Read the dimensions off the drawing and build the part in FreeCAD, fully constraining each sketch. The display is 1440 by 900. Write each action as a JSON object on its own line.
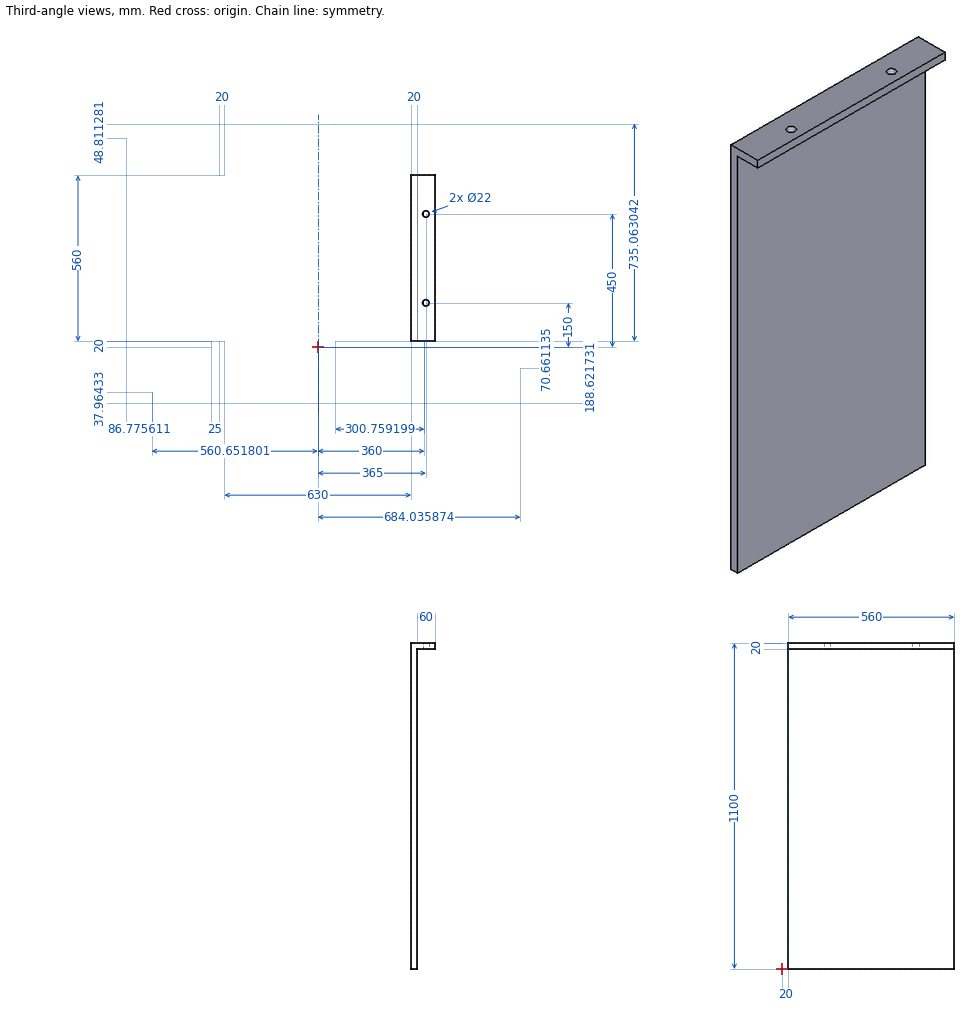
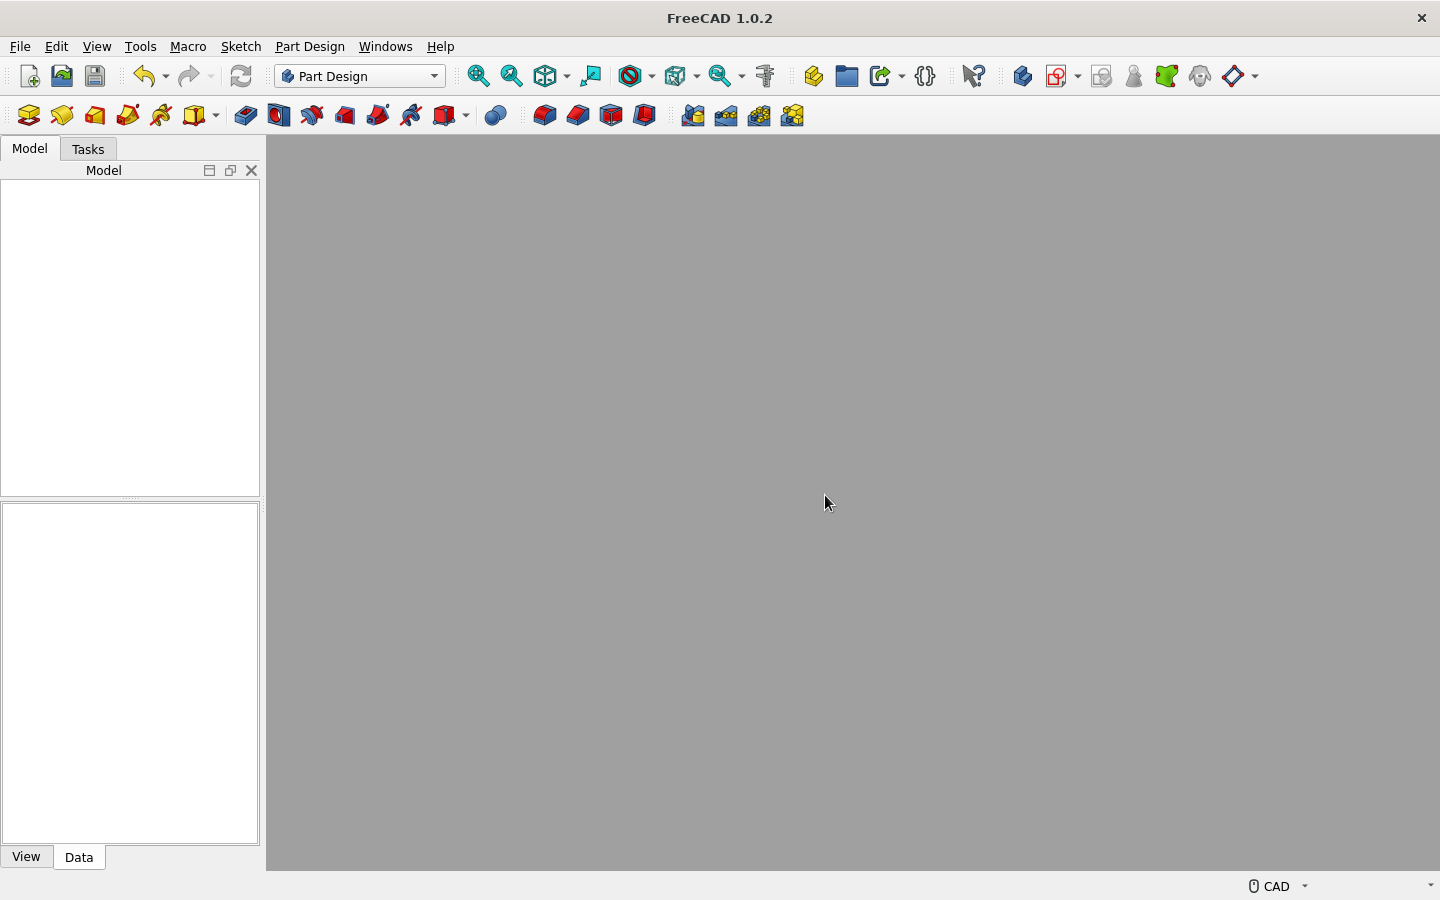
{"action": "left_click", "coordinate": [29, 76]}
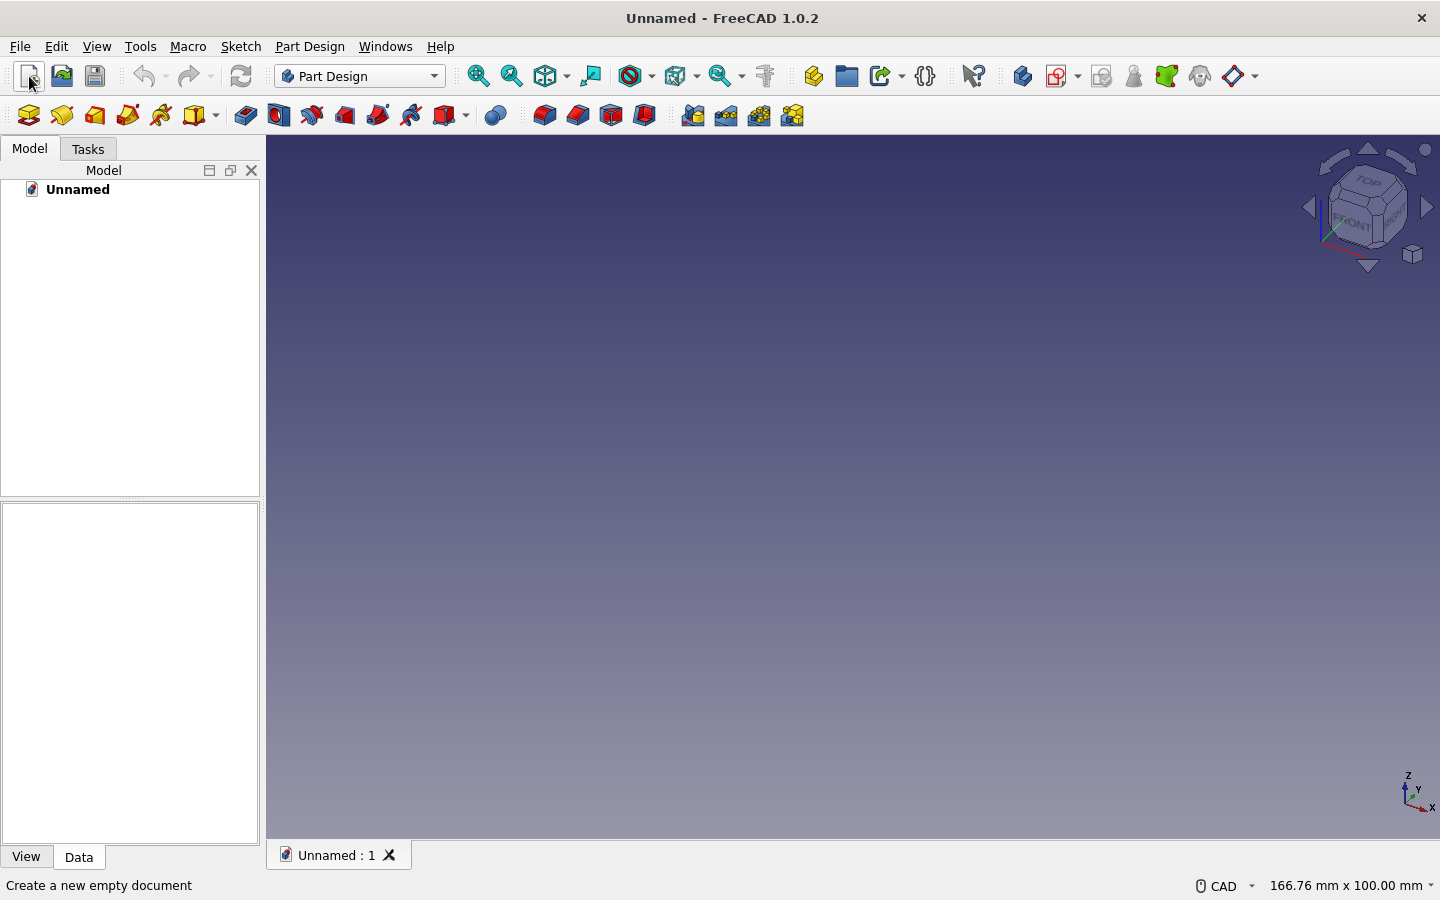
{"action": "left_click", "coordinate": [1056, 76]}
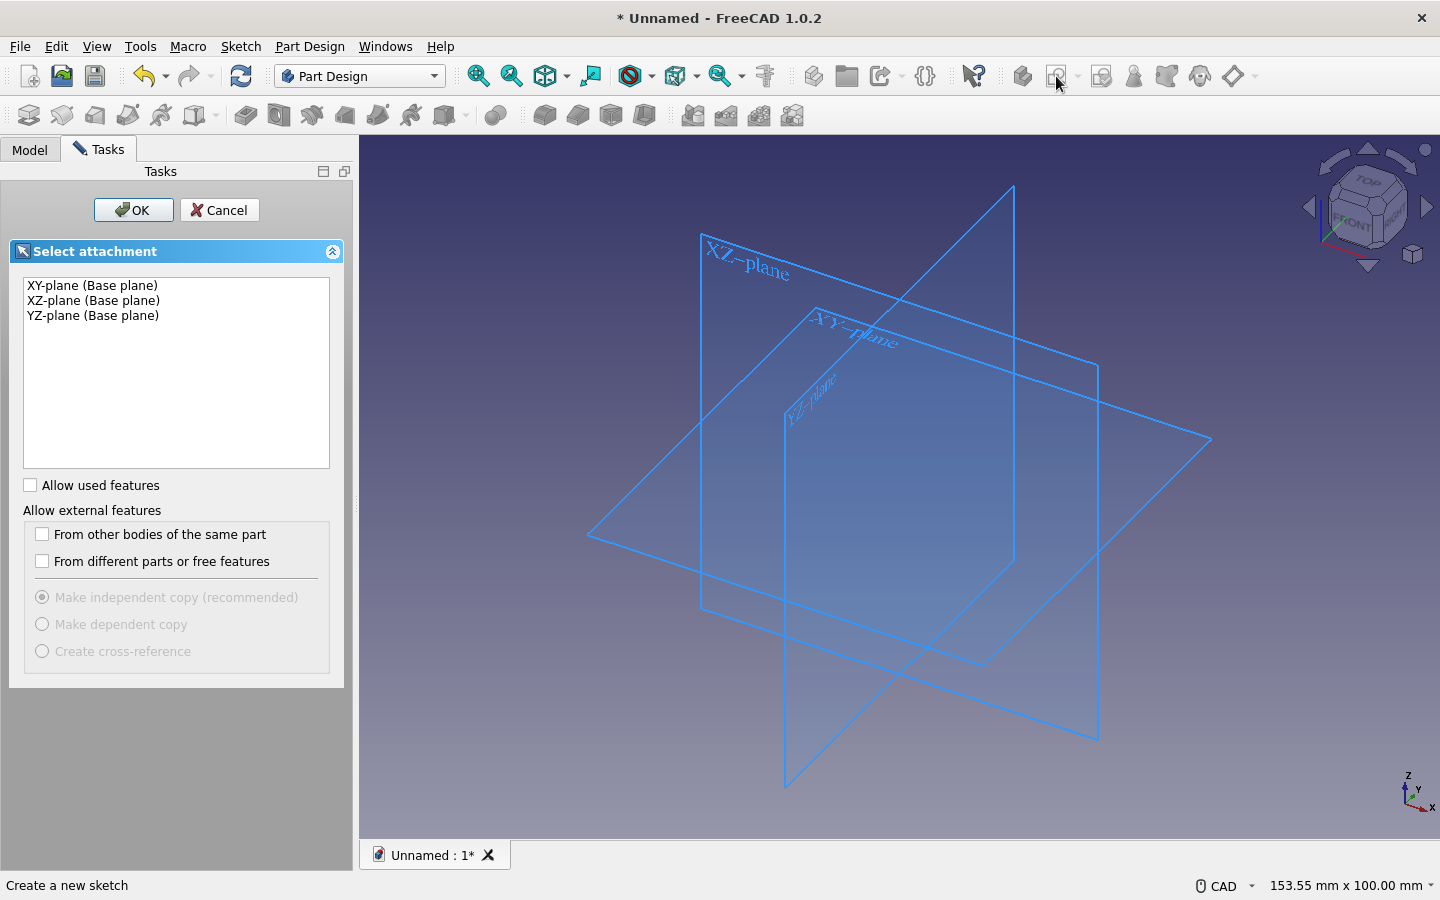
{"action": "left_click", "coordinate": [84, 286]}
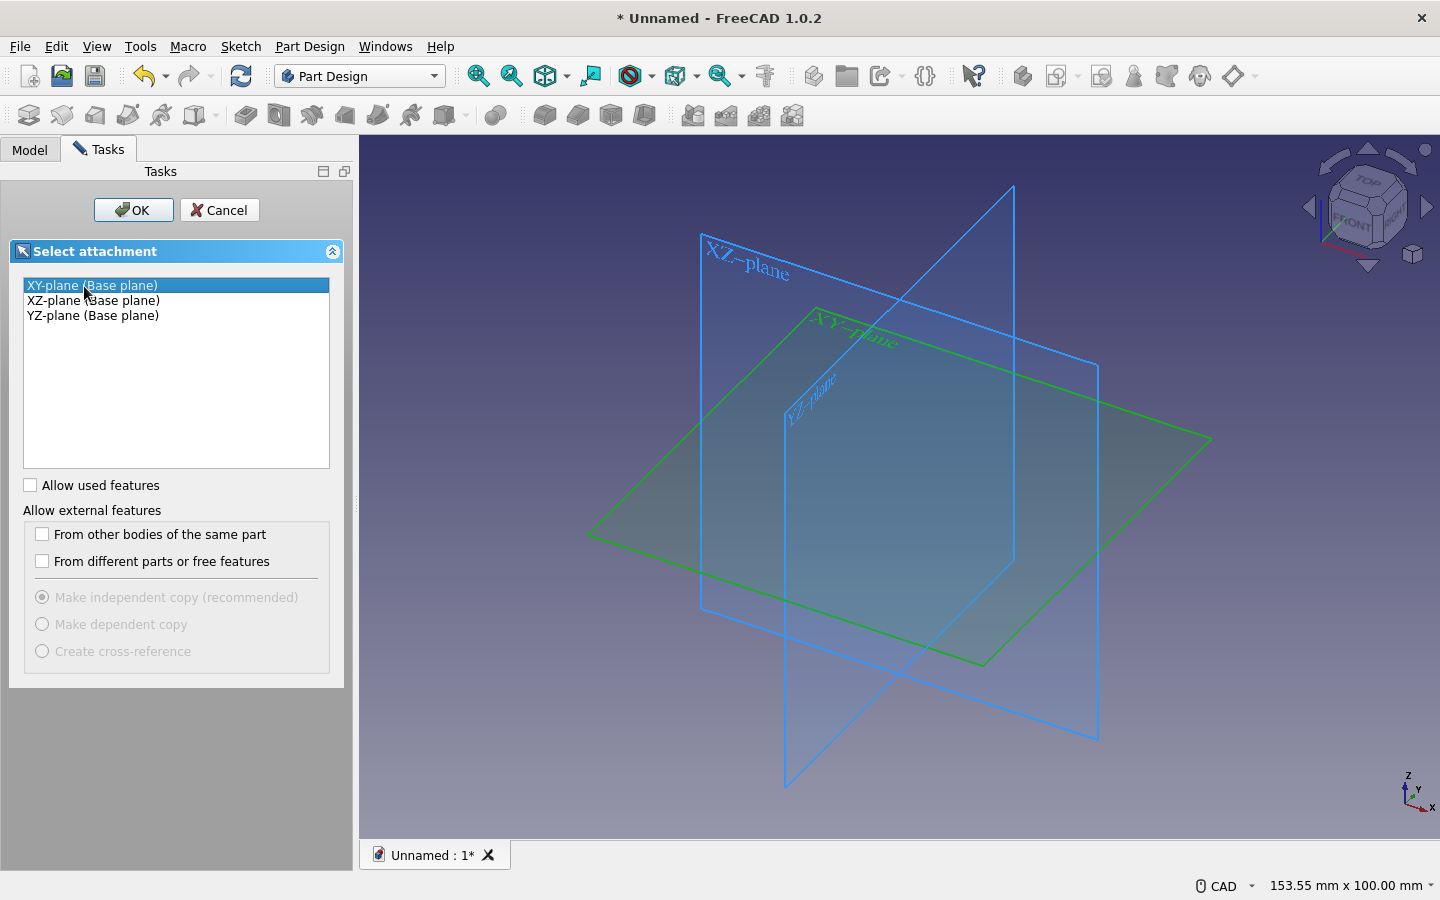
{"action": "left_click", "coordinate": [134, 210]}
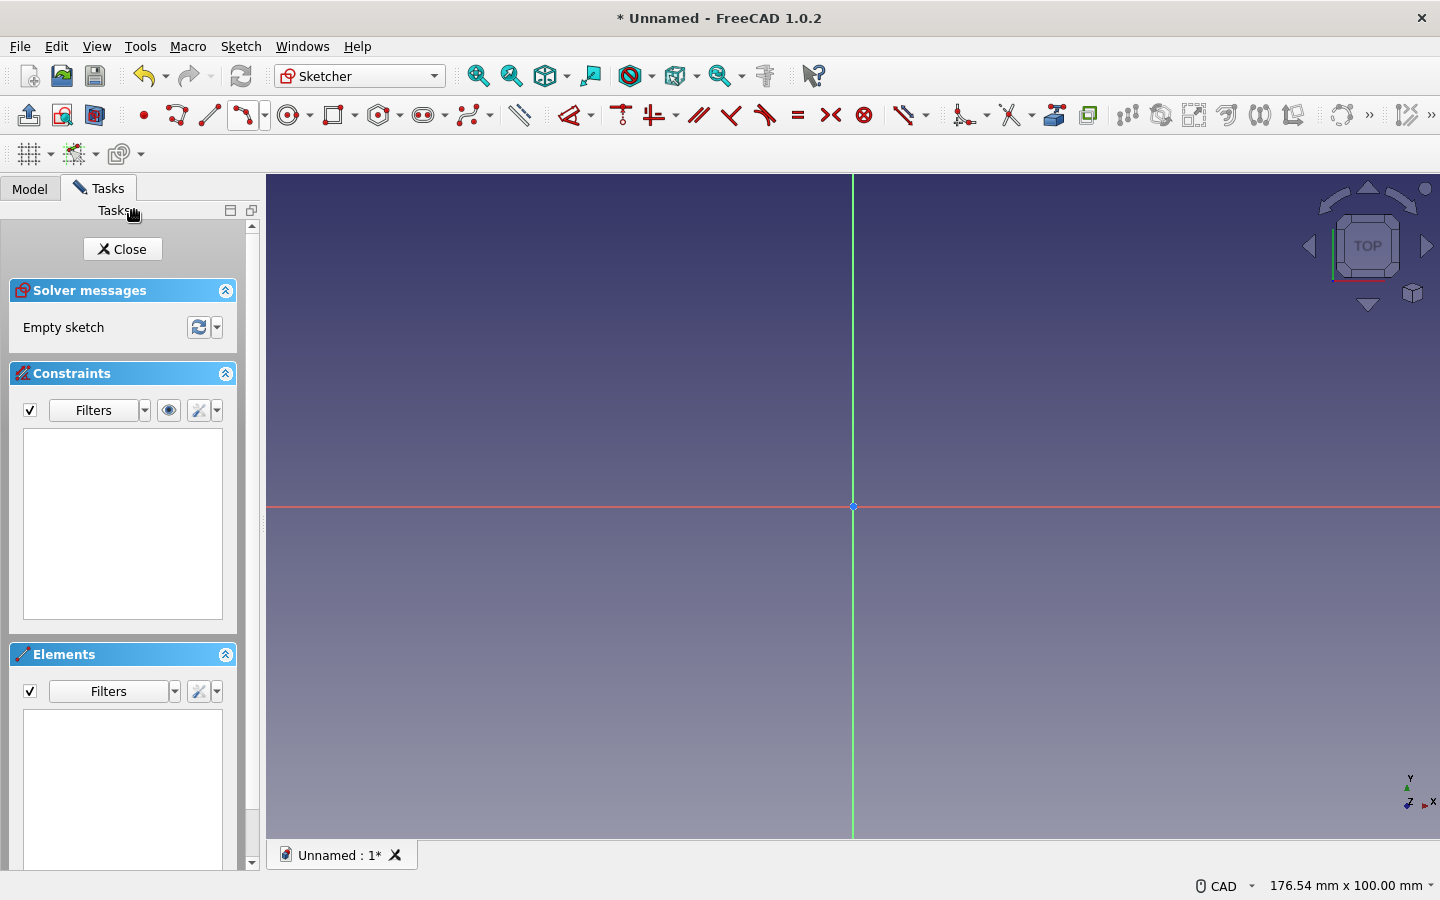
{"action": "scroll", "coordinate": [776, 747], "scroll_direction": "down", "scroll_amount": 11}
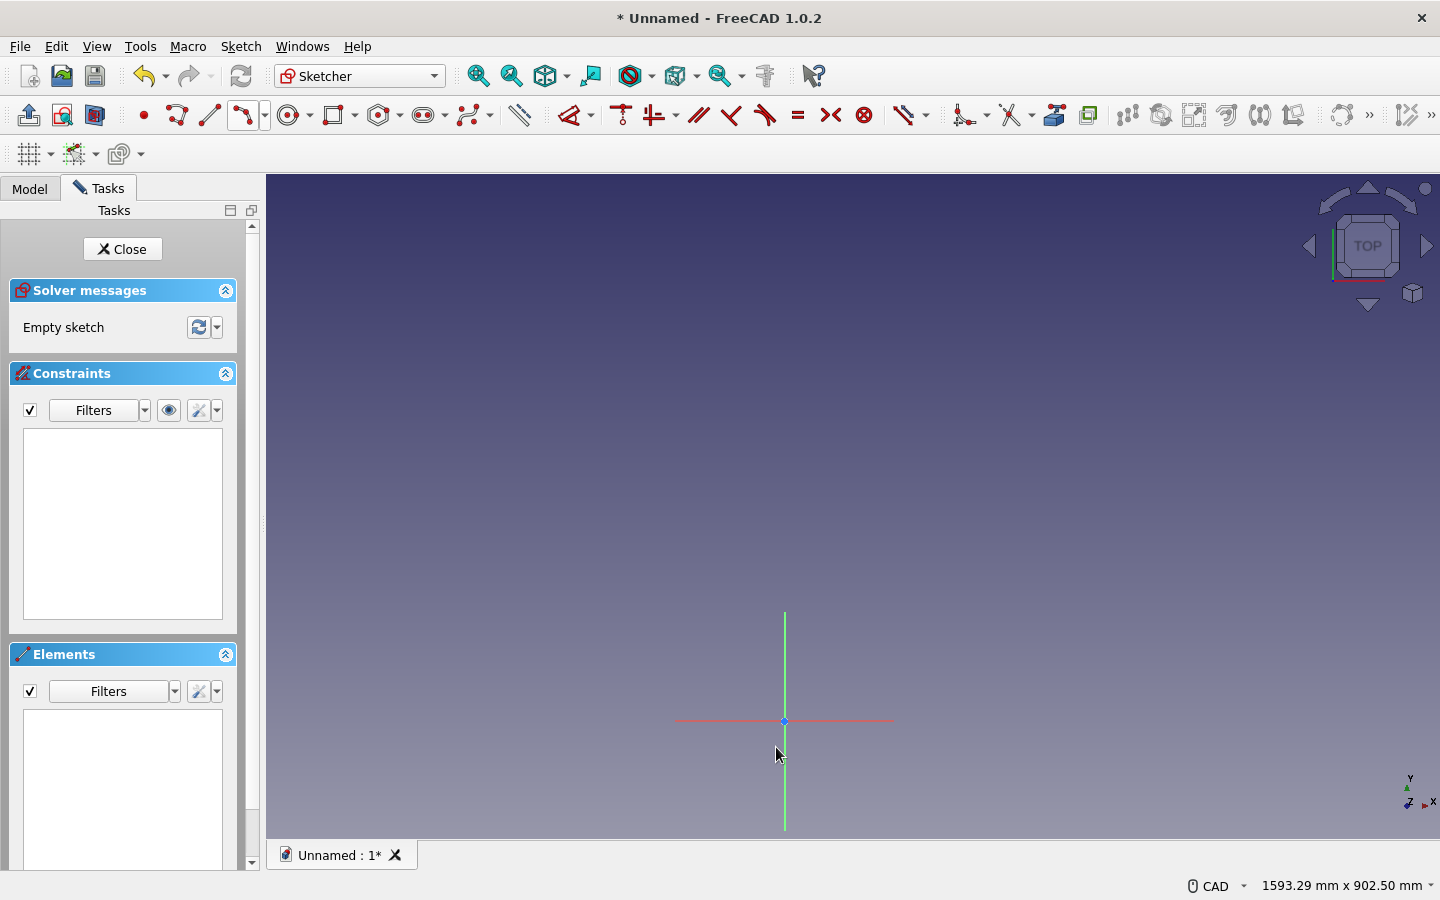
{"action": "left_click", "coordinate": [177, 116]}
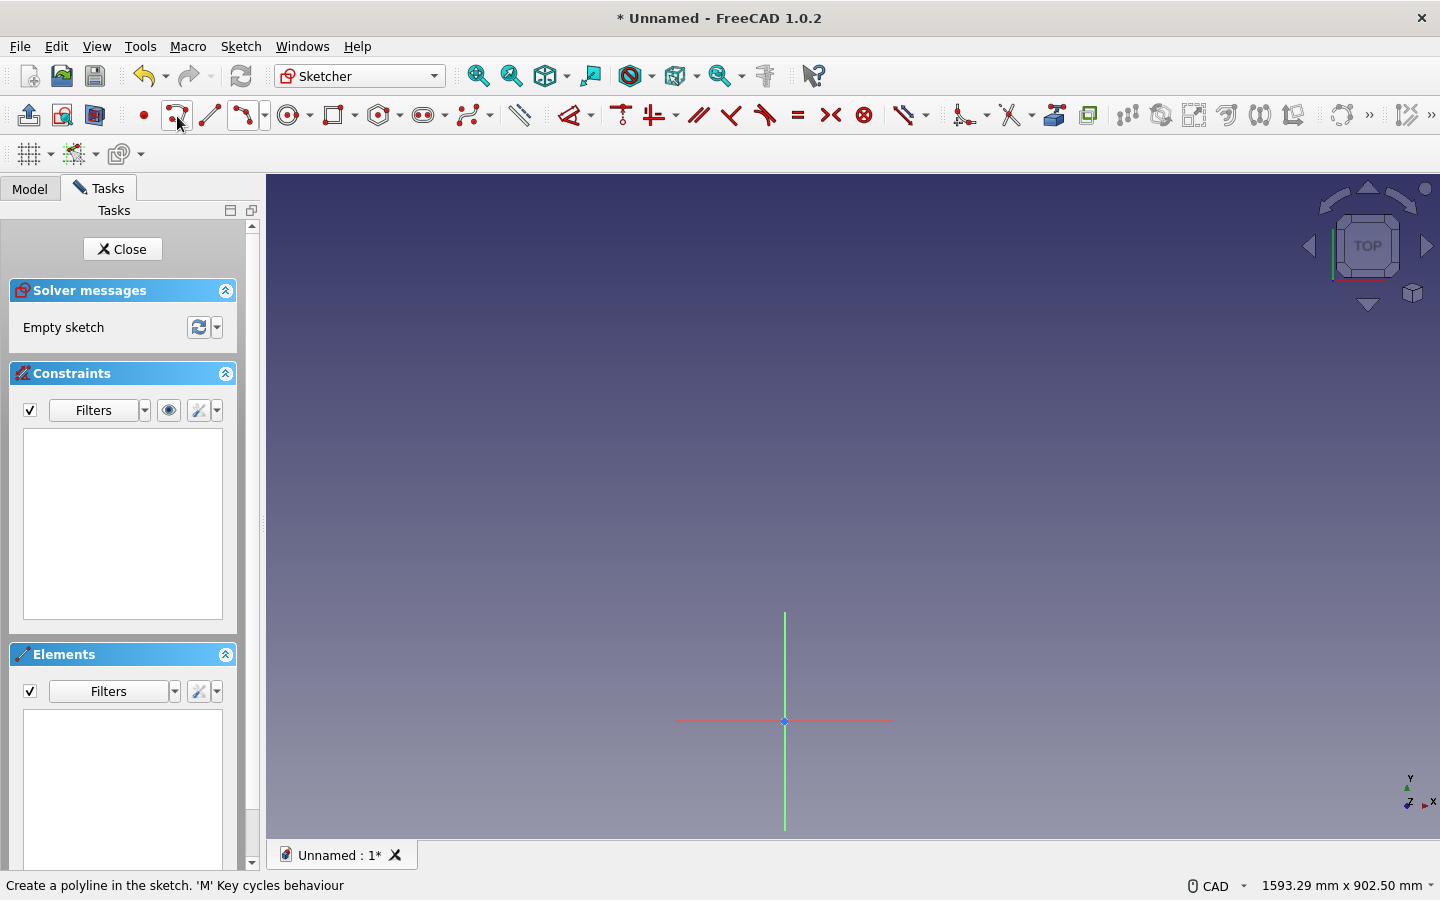
{"action": "left_click", "coordinate": [1017, 706]}
{"action": "left_click", "coordinate": [553, 706]}
{"action": "left_click", "coordinate": [553, 294]}
{"action": "left_click", "coordinate": [538, 294]}
{"action": "left_click", "coordinate": [538, 706]}
{"action": "left_click", "coordinate": [520, 706]}
{"action": "left_click", "coordinate": [520, 721]}
{"action": "left_click", "coordinate": [1050, 712]}
{"action": "left_click", "coordinate": [1050, 706]}
{"action": "left_click", "coordinate": [1032, 706]}
{"action": "left_click", "coordinate": [1032, 294]}
{"action": "left_click", "coordinate": [1017, 294]}
{"action": "left_click", "coordinate": [1017, 707]}
{"action": "key", "text": "Escape"}
{"action": "key", "text": "Escape"}